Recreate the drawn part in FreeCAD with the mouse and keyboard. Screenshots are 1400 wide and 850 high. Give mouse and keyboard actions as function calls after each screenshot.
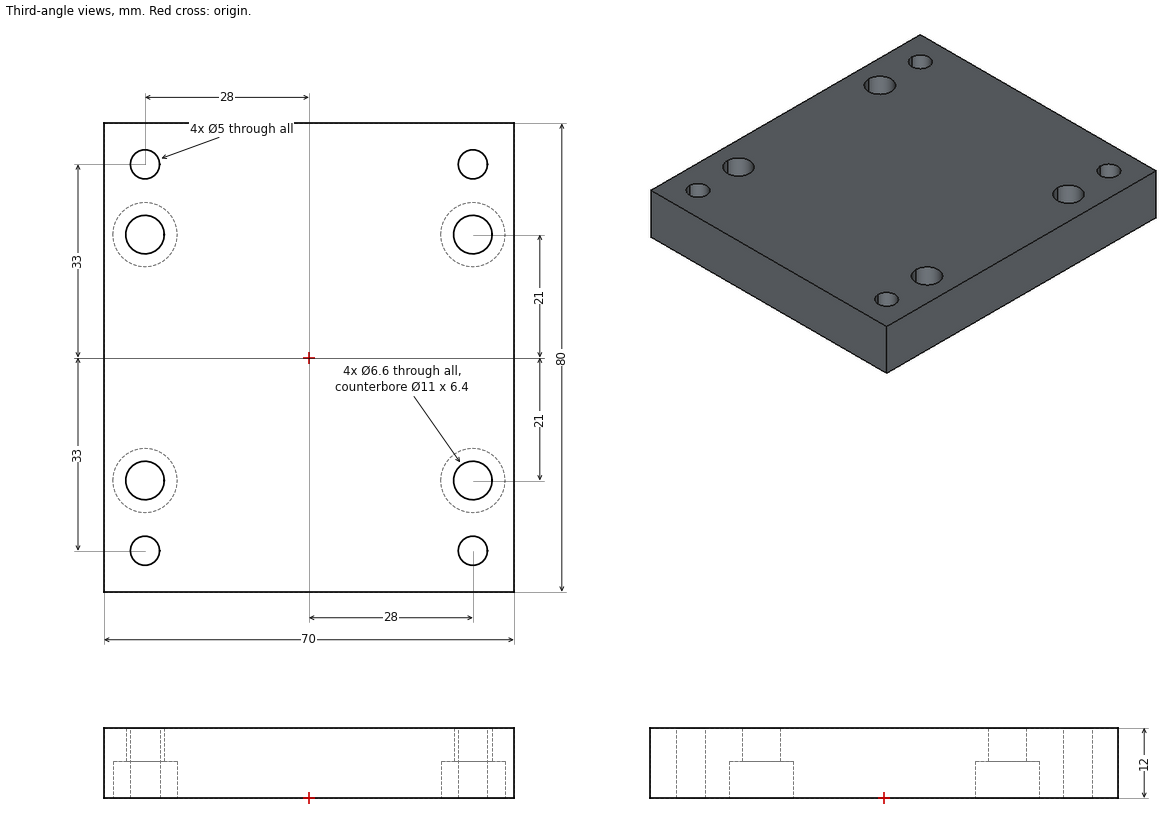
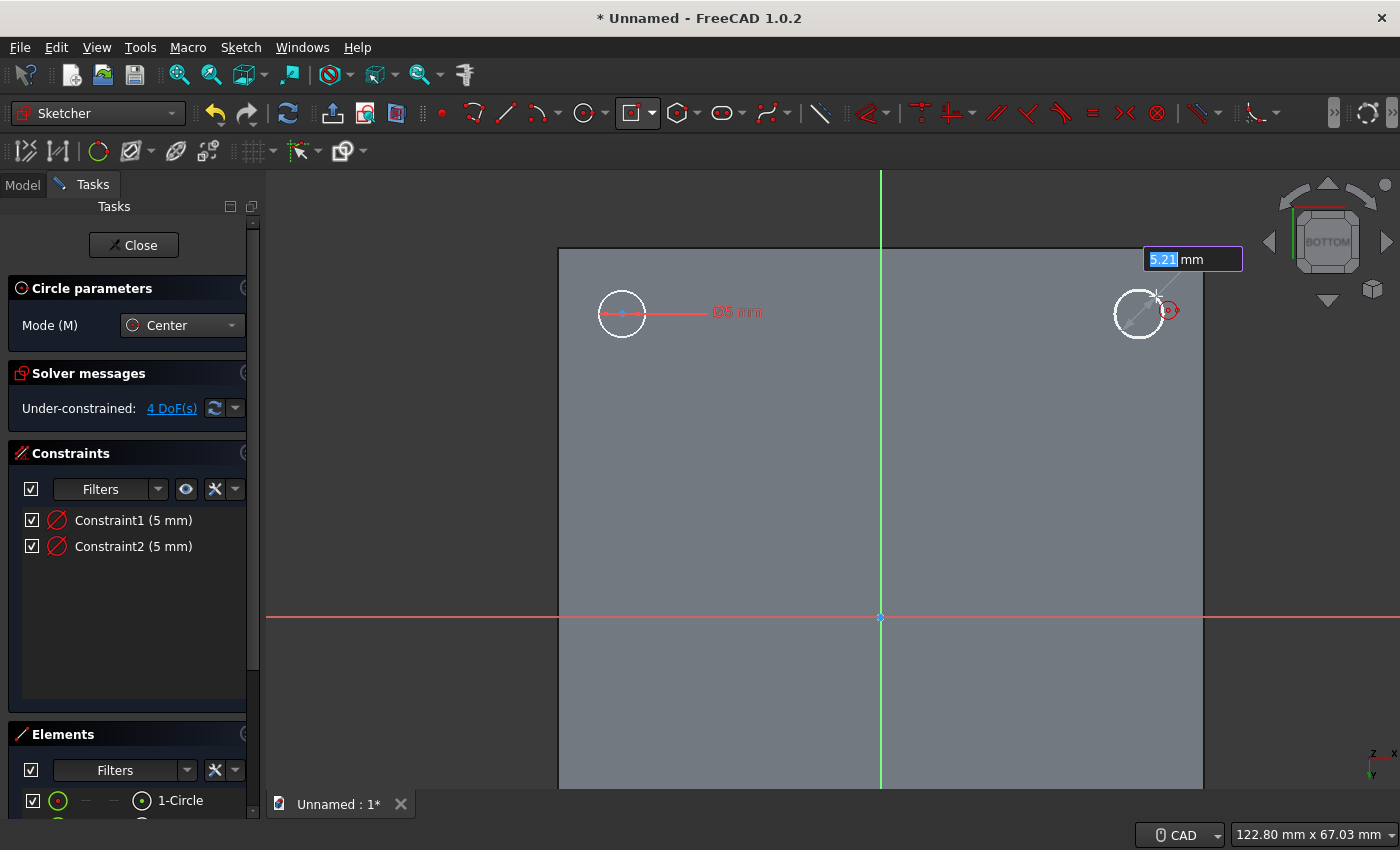
text(5)
key(Return)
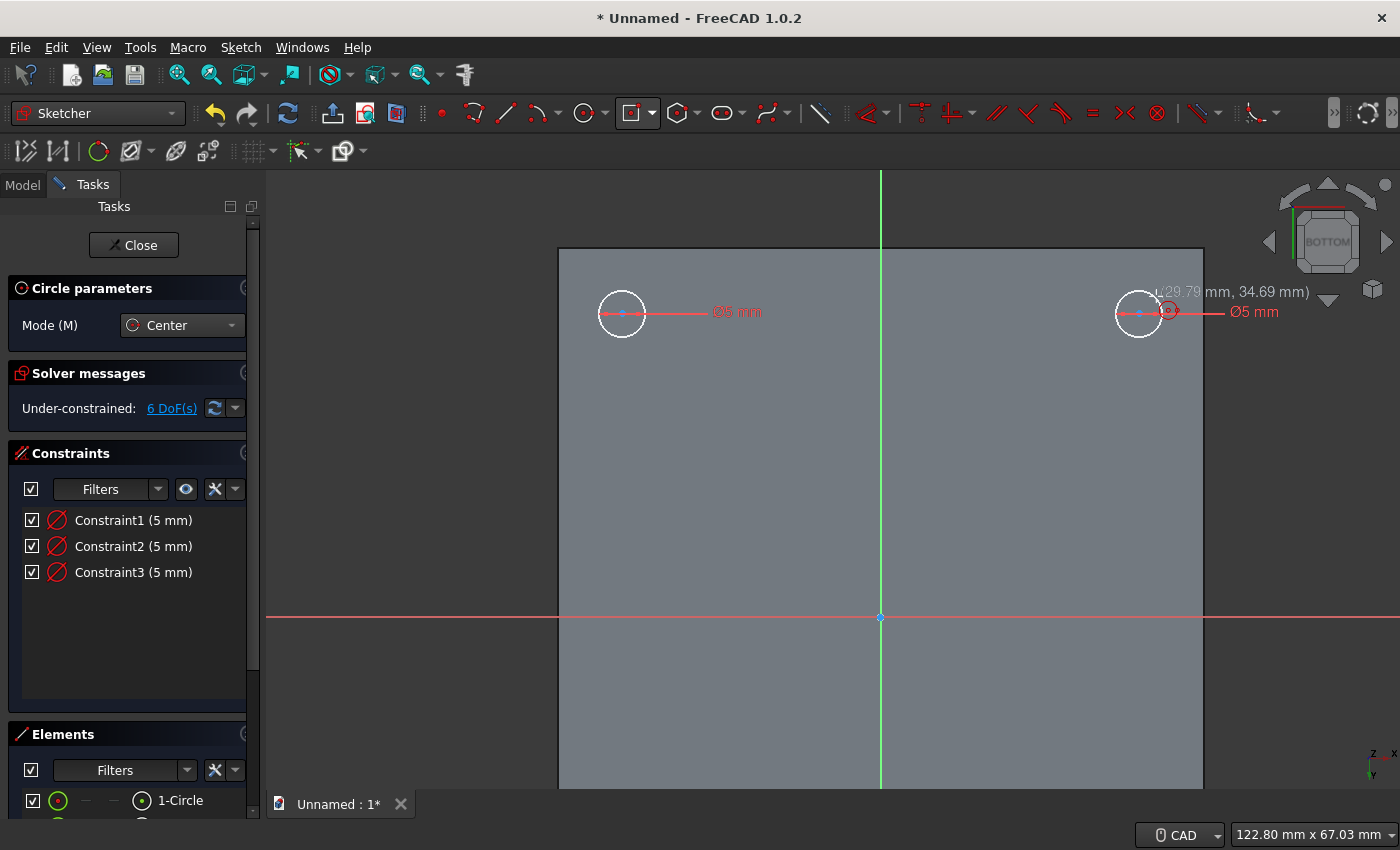
scroll(623, 312, down, 3)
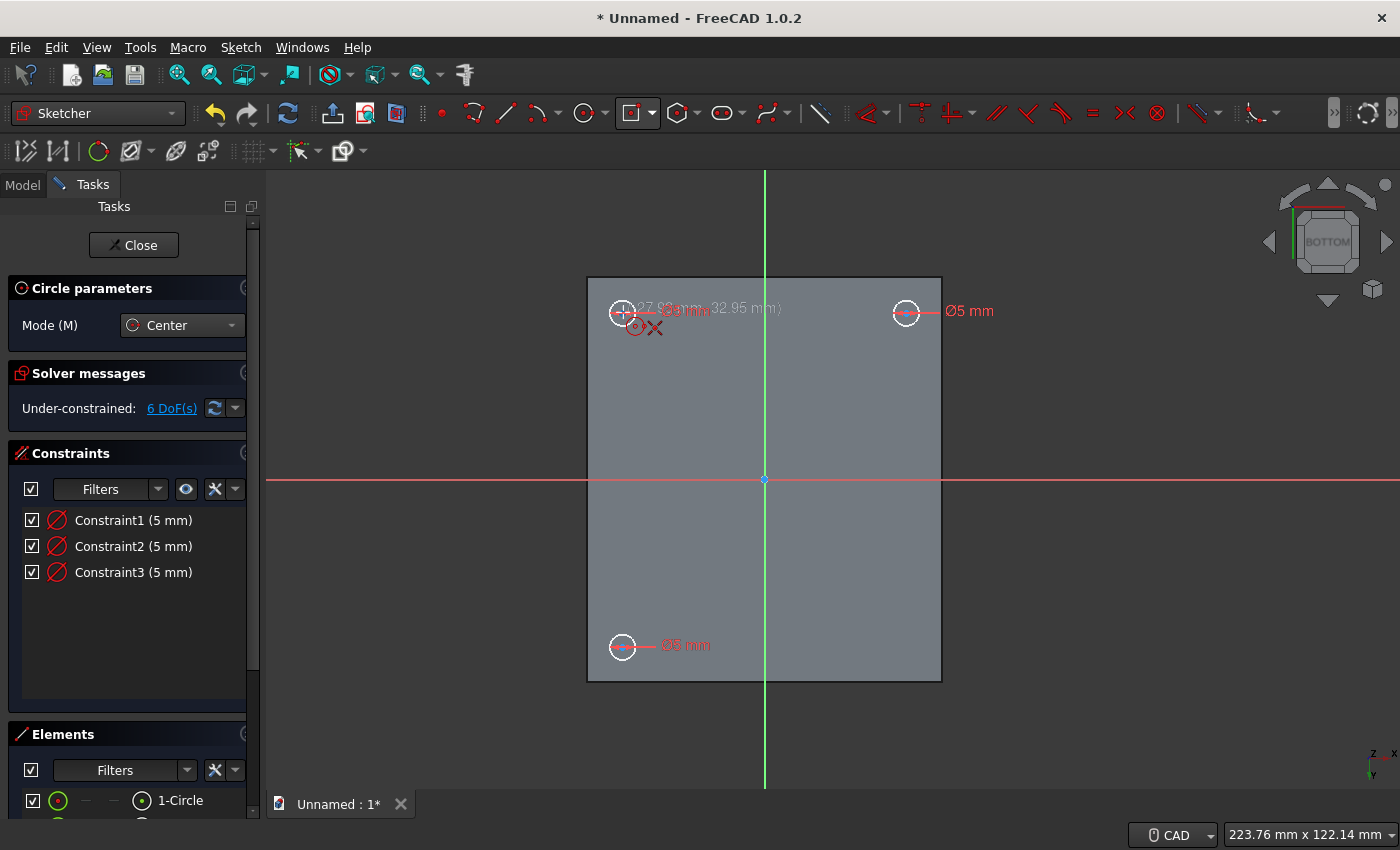
scroll(907, 647, up, 3)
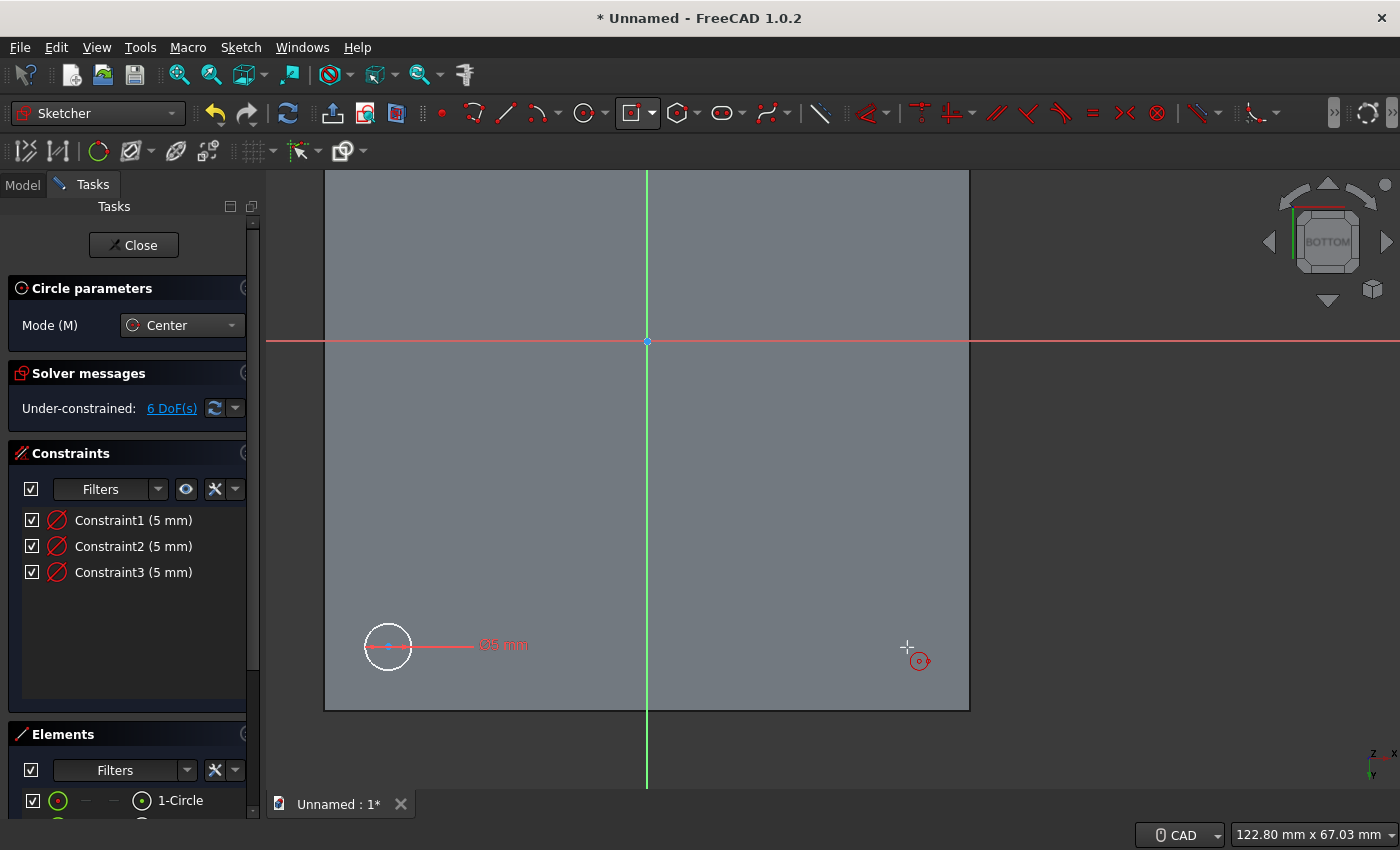
click(906, 646)
move(922, 630)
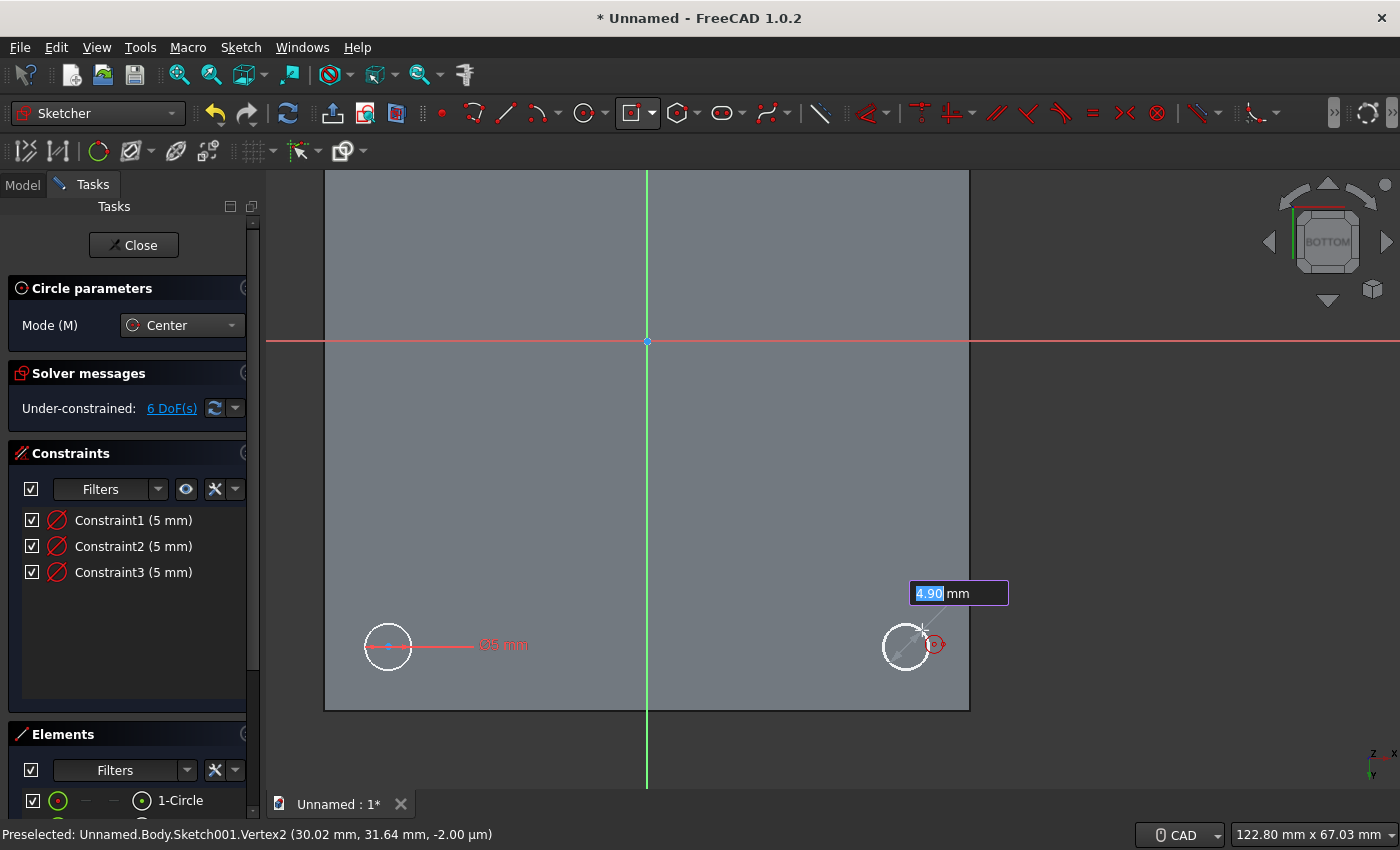
text(5)
key(Return)
key(Escape)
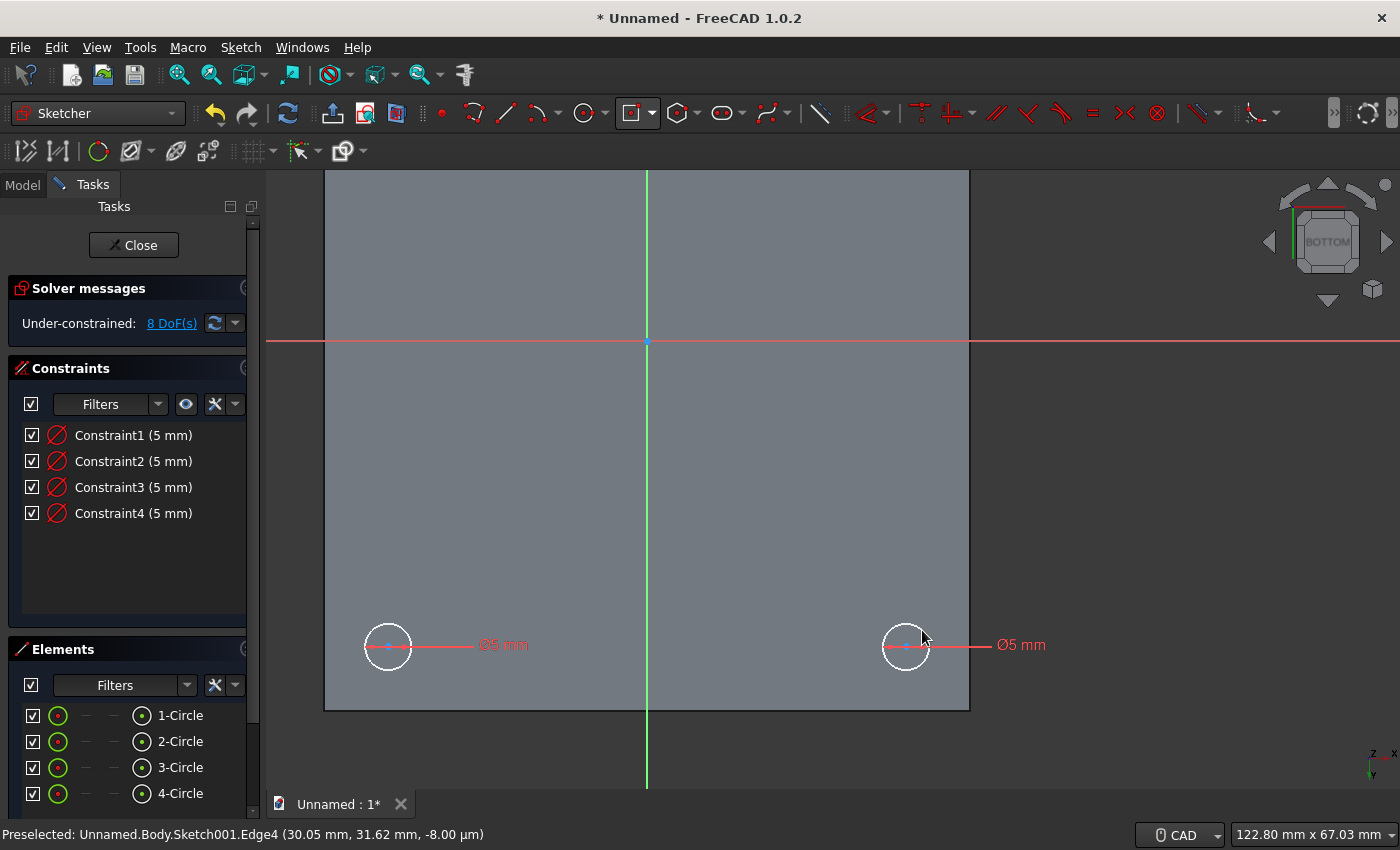
click(388, 647)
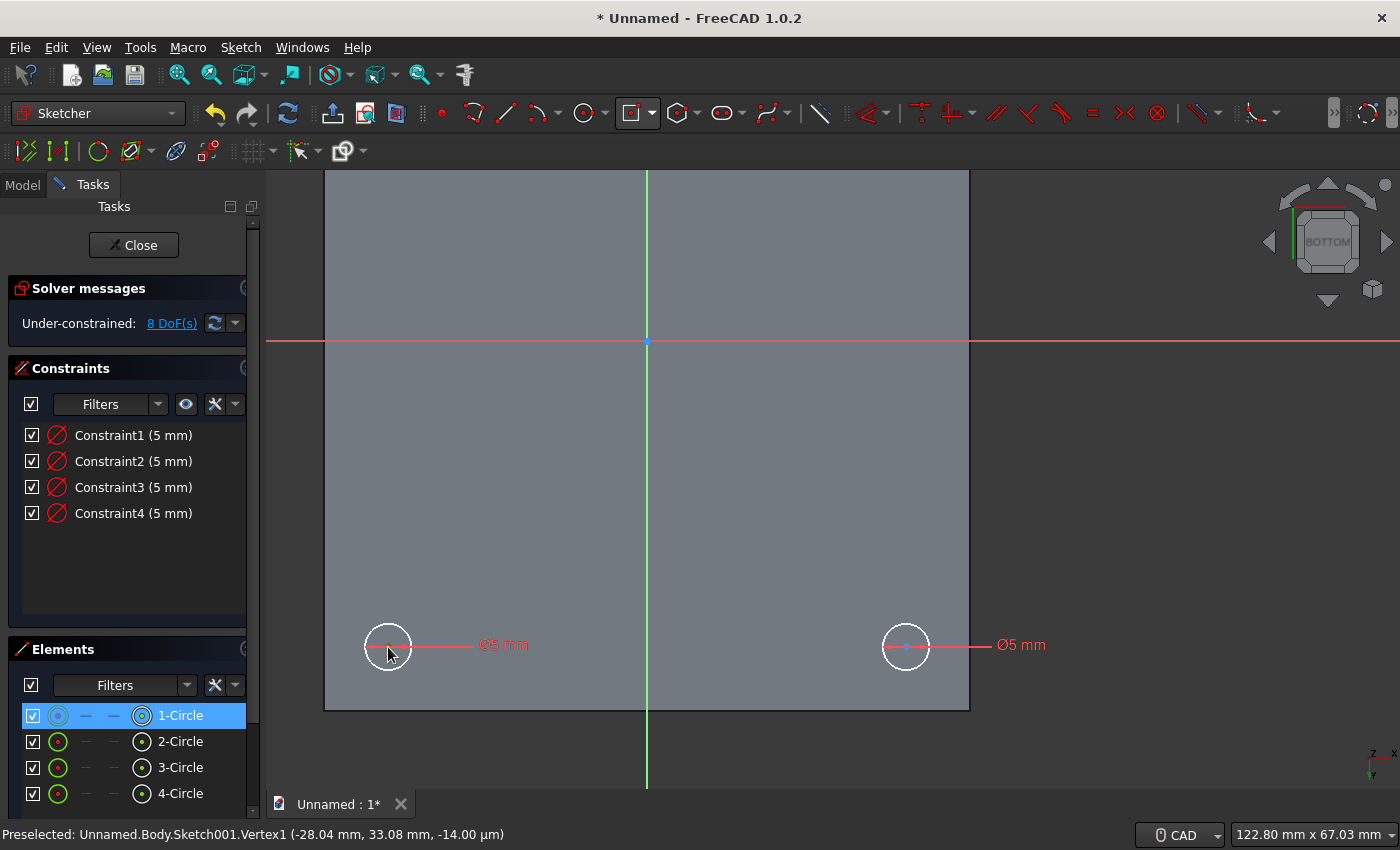
scroll(907, 647, down, 3)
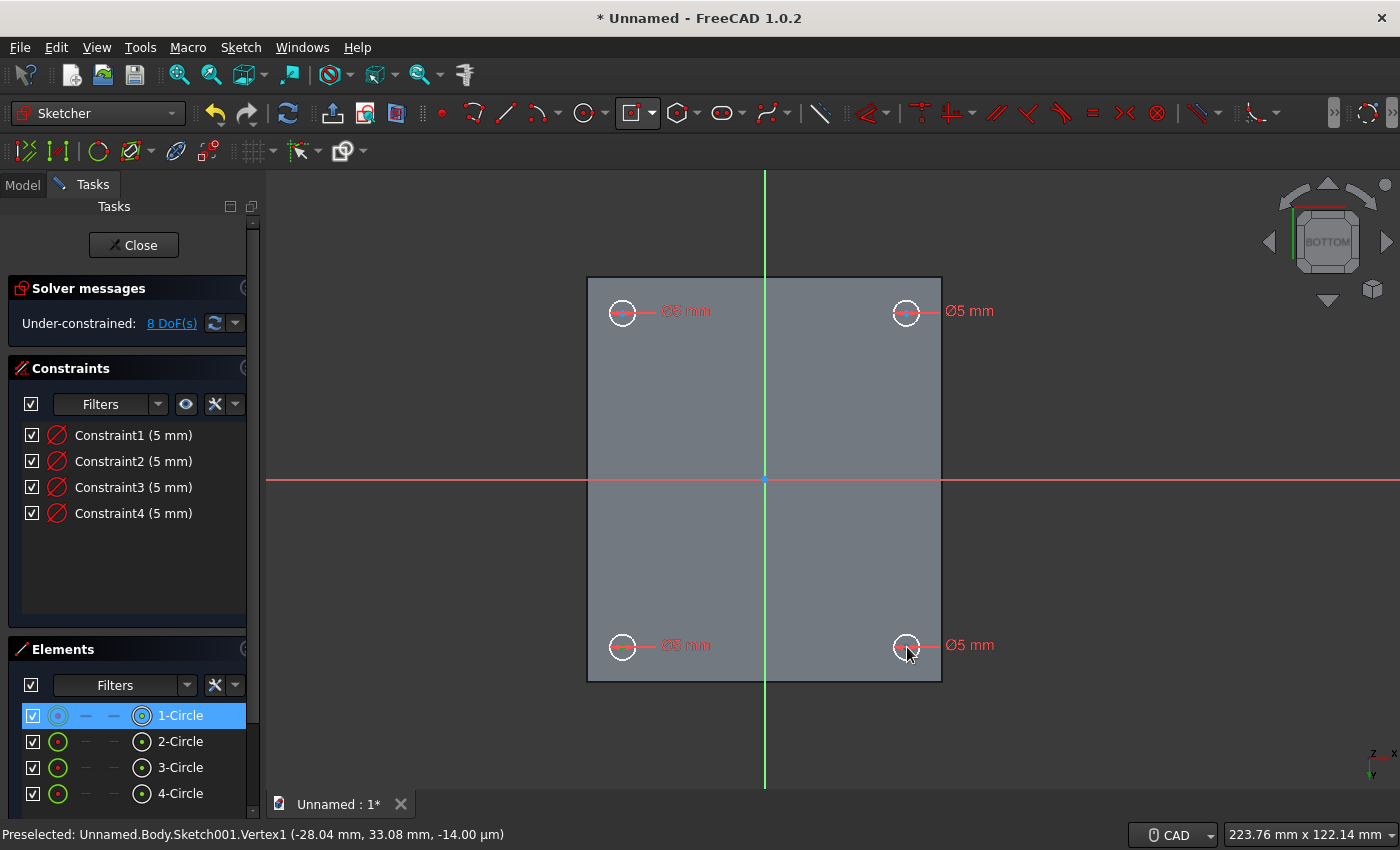
click(623, 313)